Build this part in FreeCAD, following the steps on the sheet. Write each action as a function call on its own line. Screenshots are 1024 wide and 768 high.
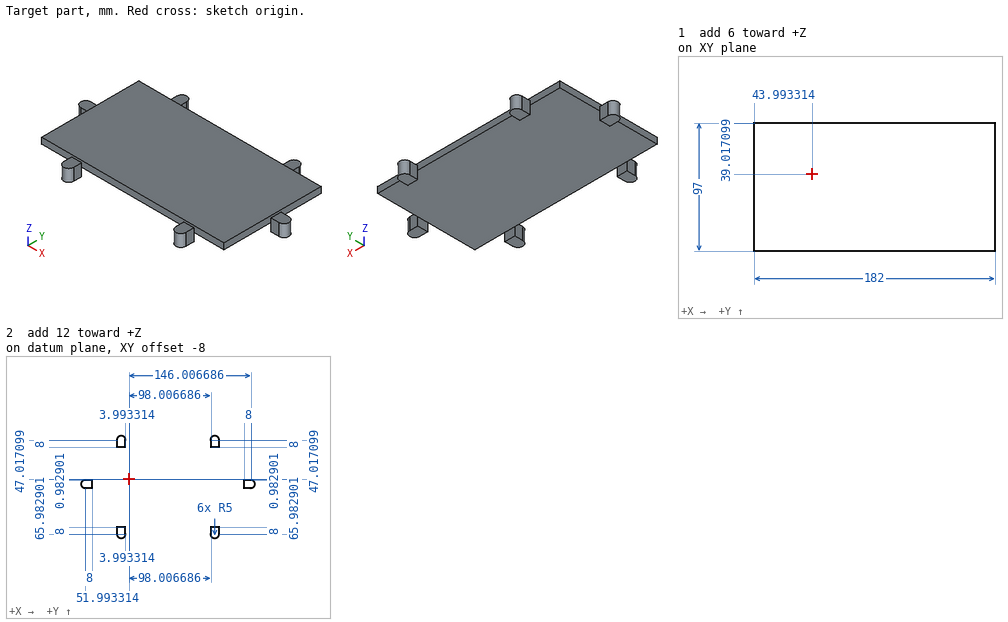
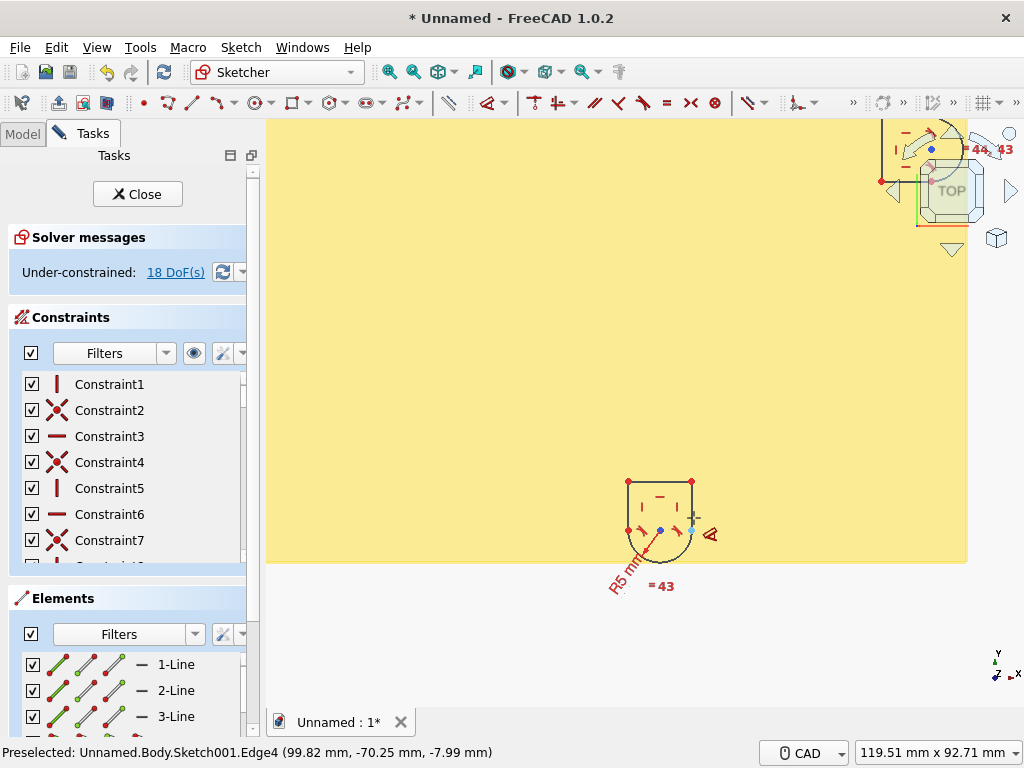
click(692, 516)
click(726, 506)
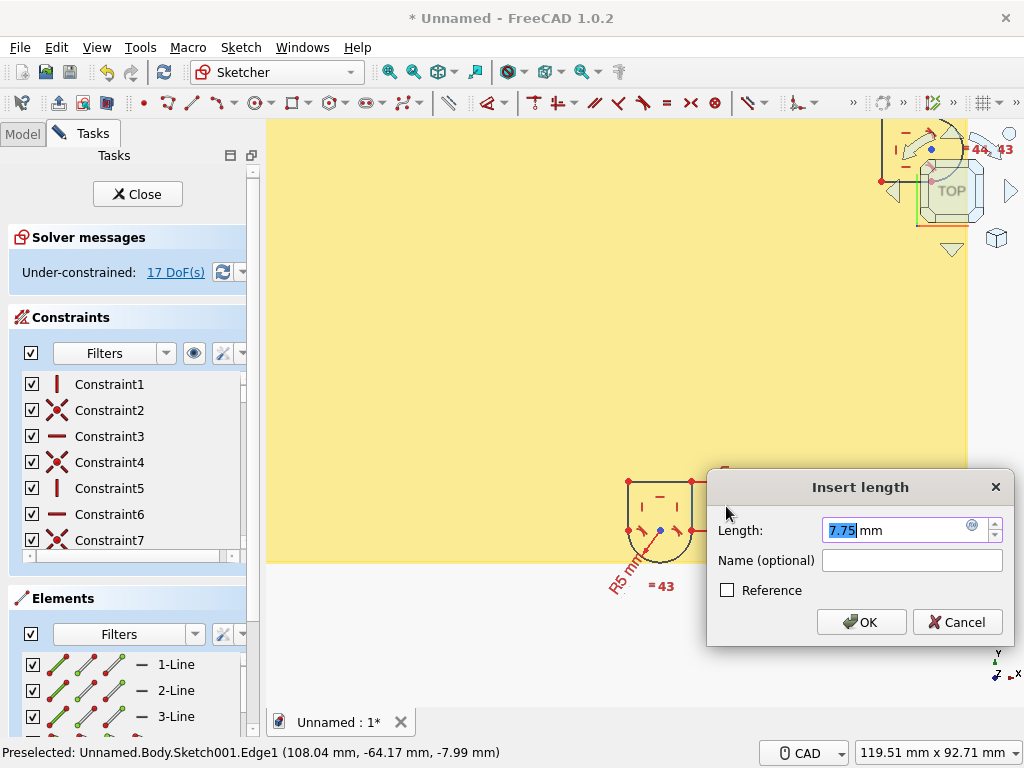
text(8)
key(Return)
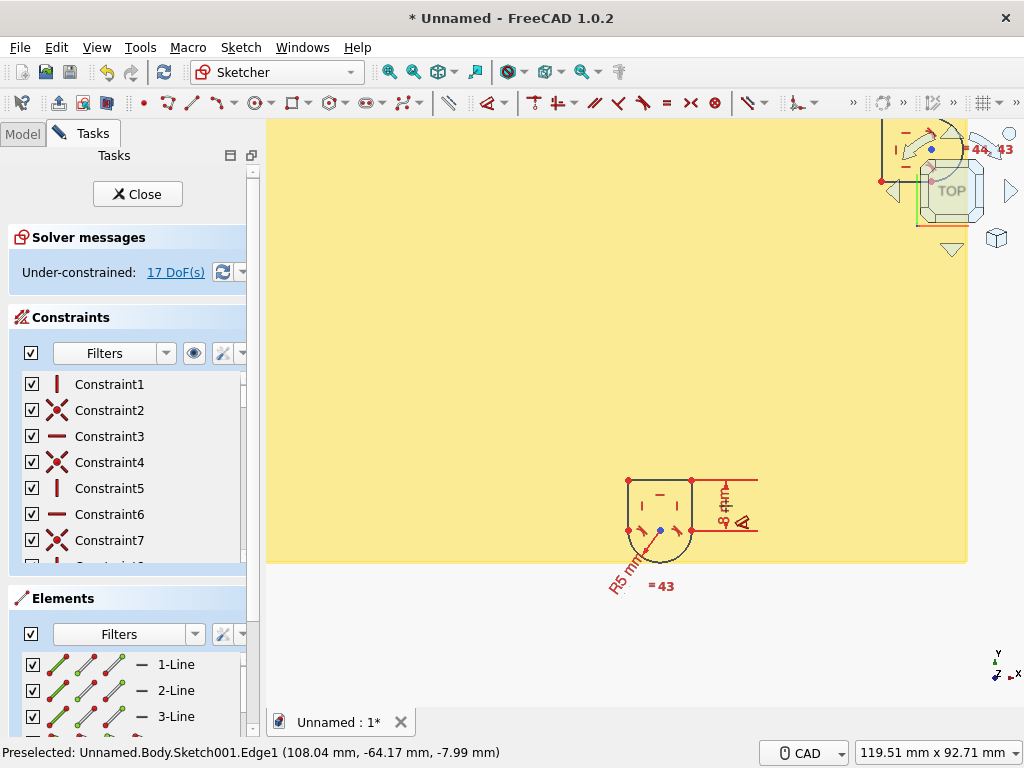
scroll(694, 518, down, 6)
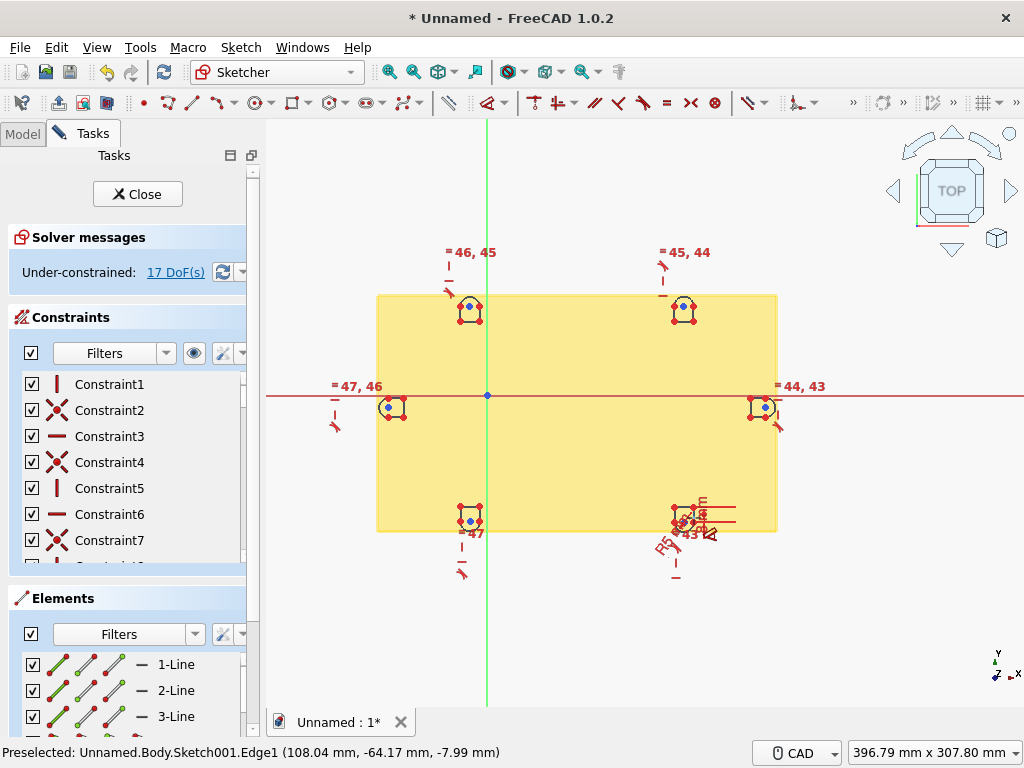
scroll(761, 398, up, 9)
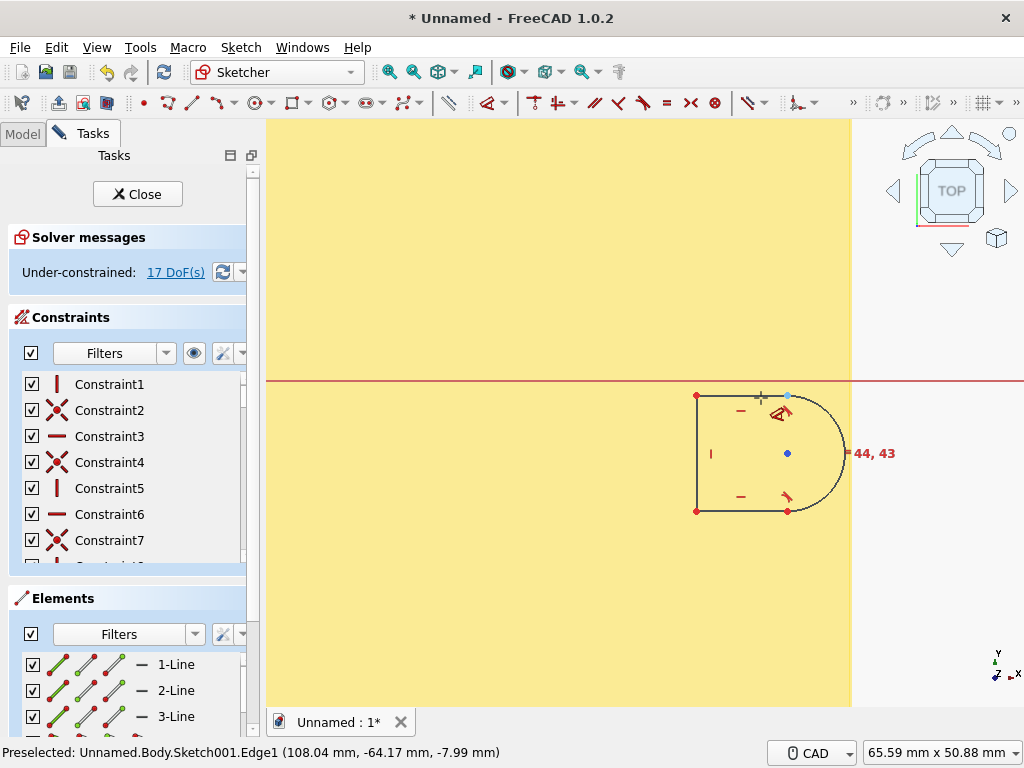
click(760, 396)
click(742, 362)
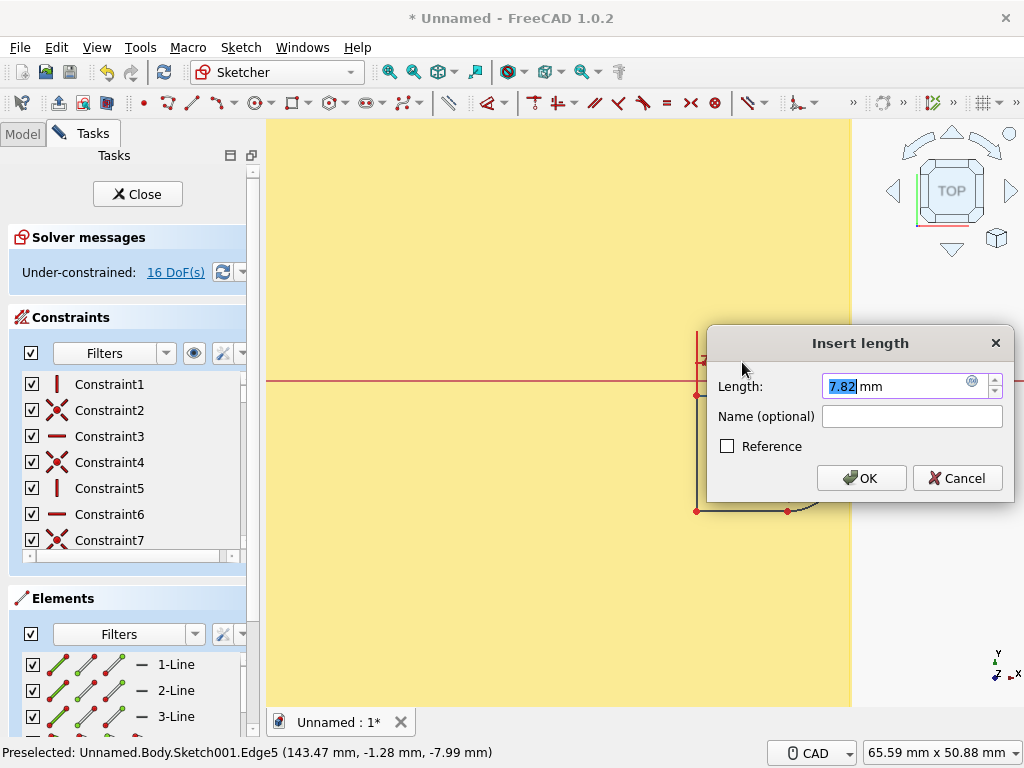
text(8)
key(Return)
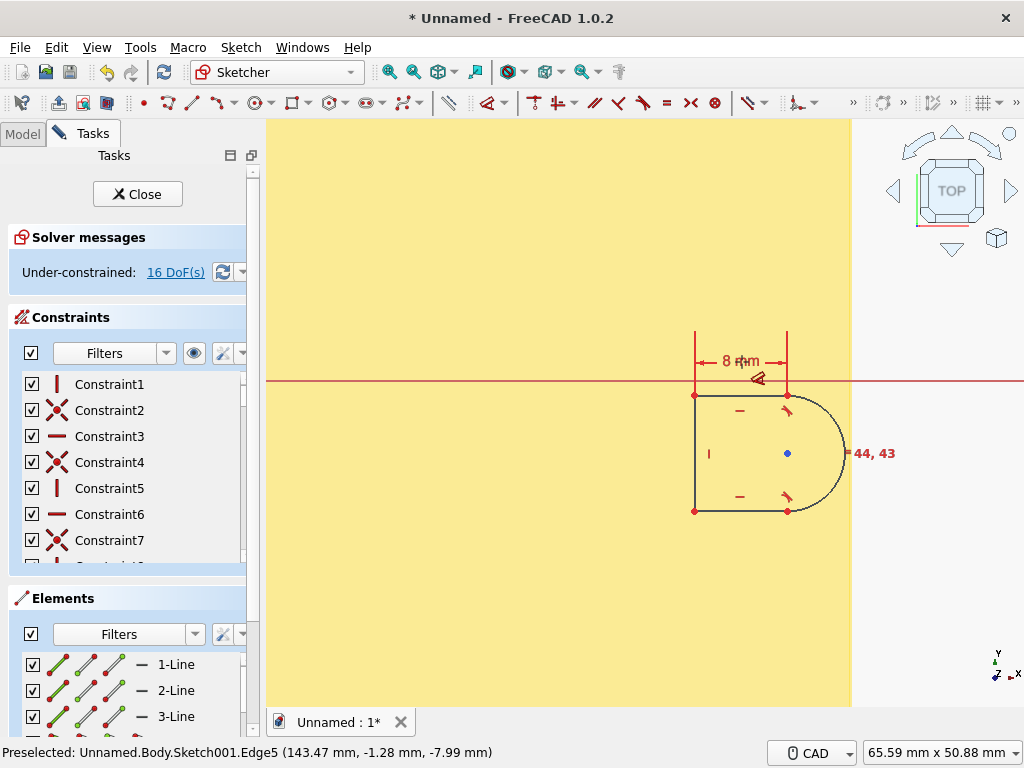
scroll(761, 398, down, 9)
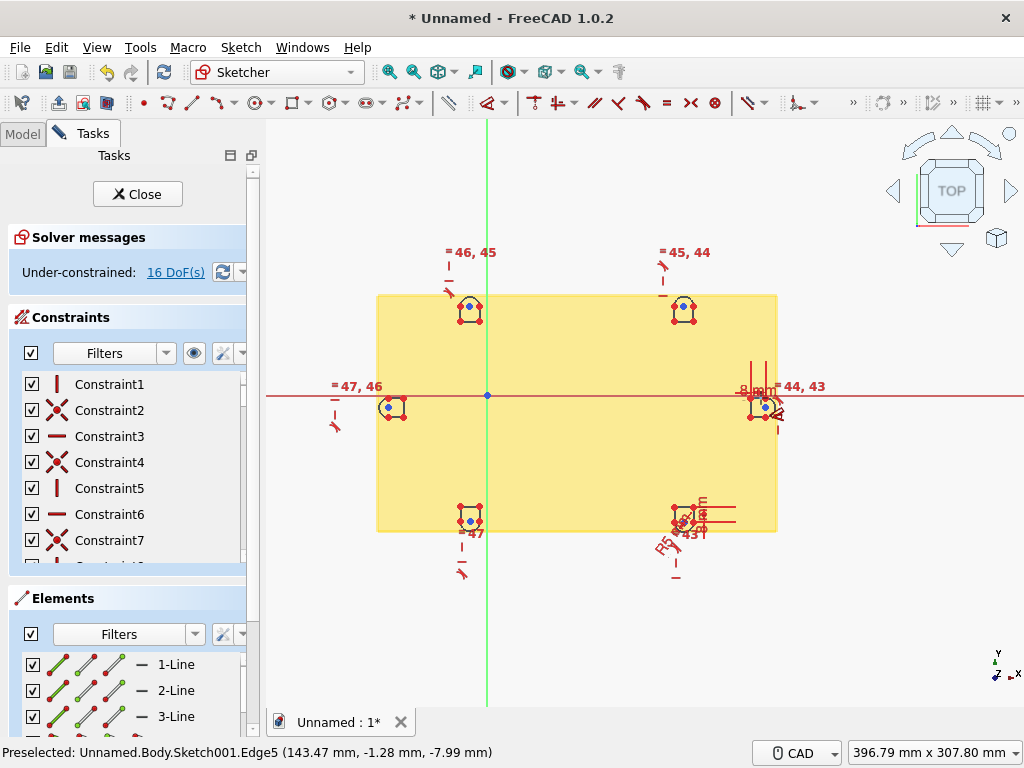
scroll(674, 311, up, 6)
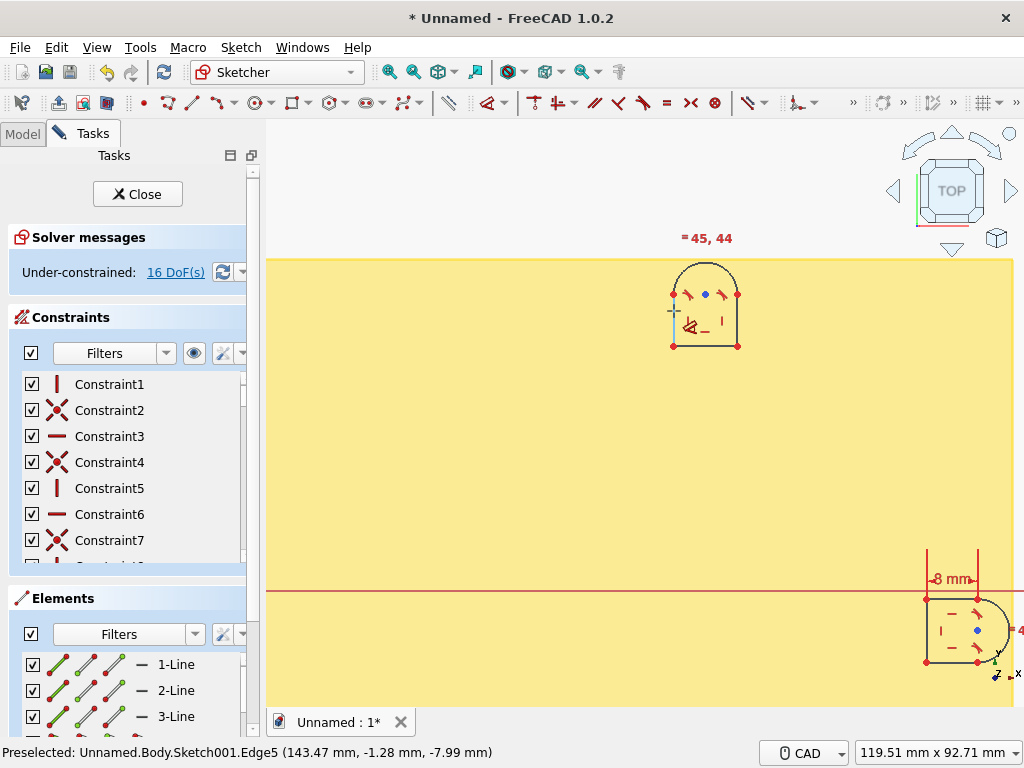
click(674, 310)
click(708, 320)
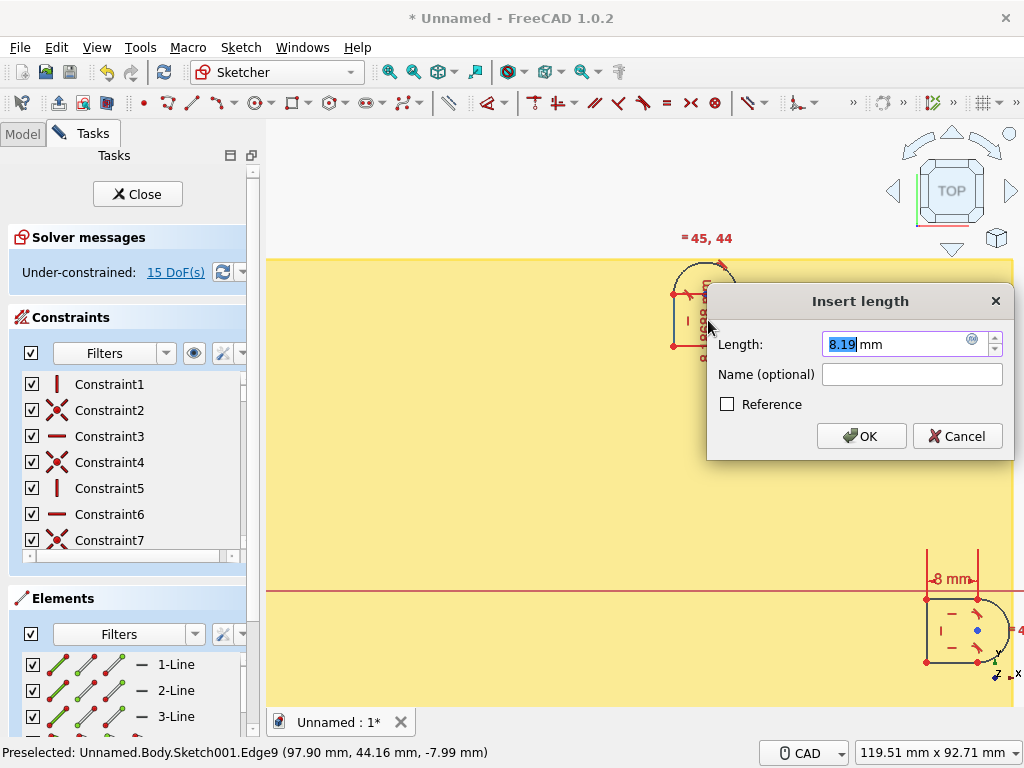
text(8)
key(Return)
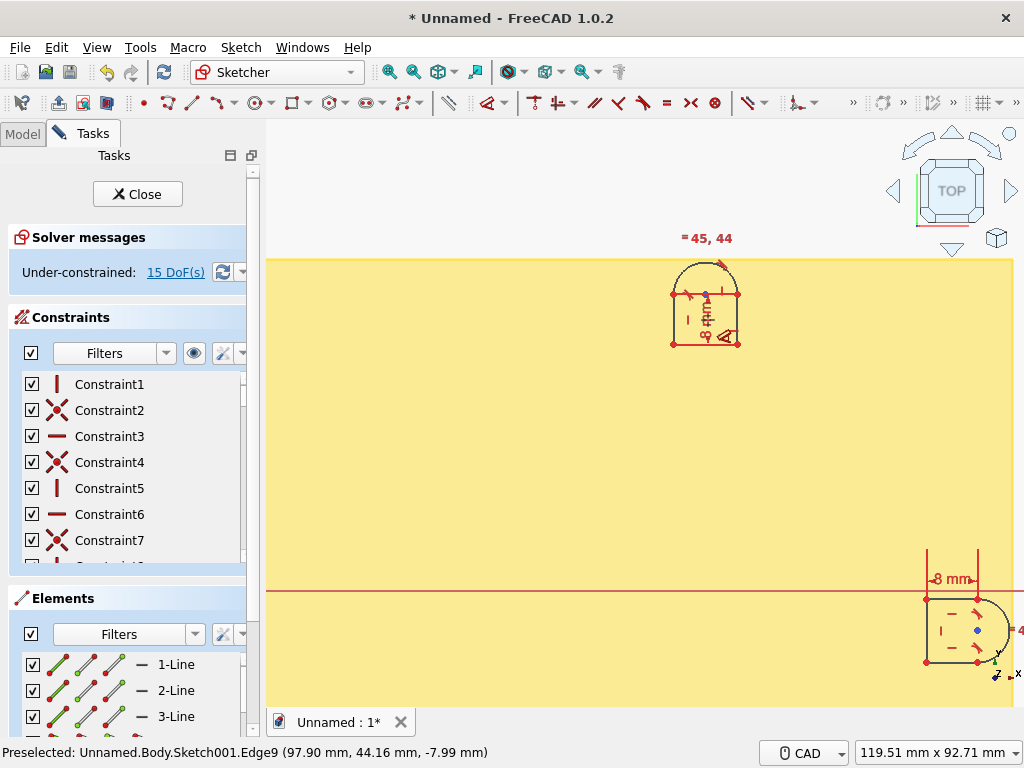
scroll(674, 310, down, 6)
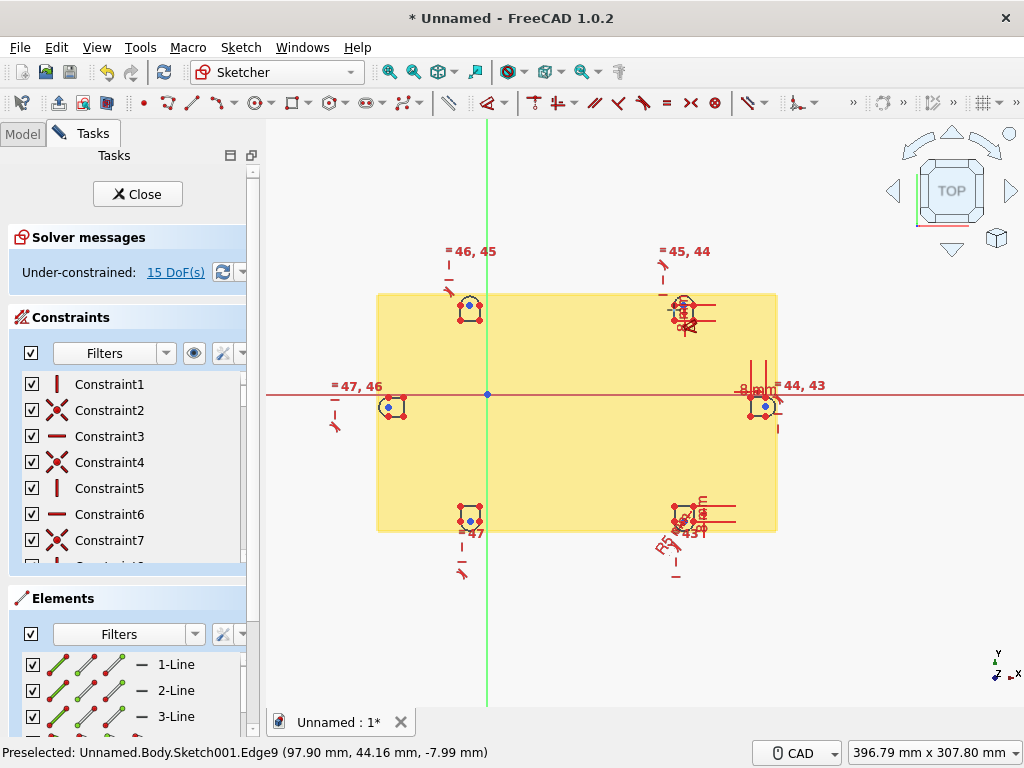
scroll(460, 310, up, 6)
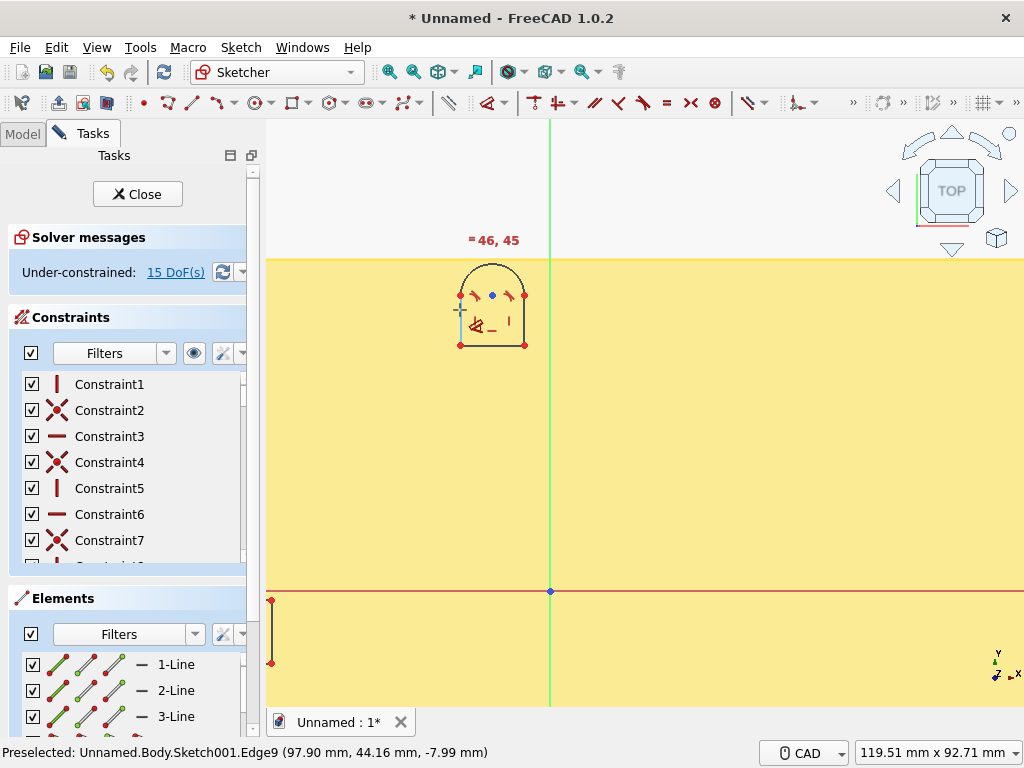
click(461, 311)
click(427, 321)